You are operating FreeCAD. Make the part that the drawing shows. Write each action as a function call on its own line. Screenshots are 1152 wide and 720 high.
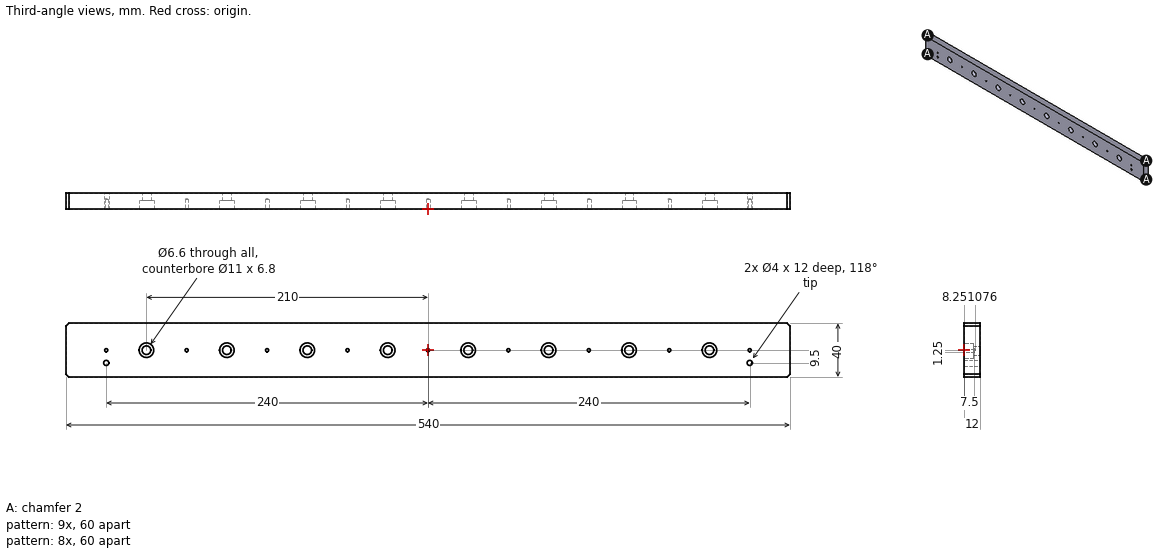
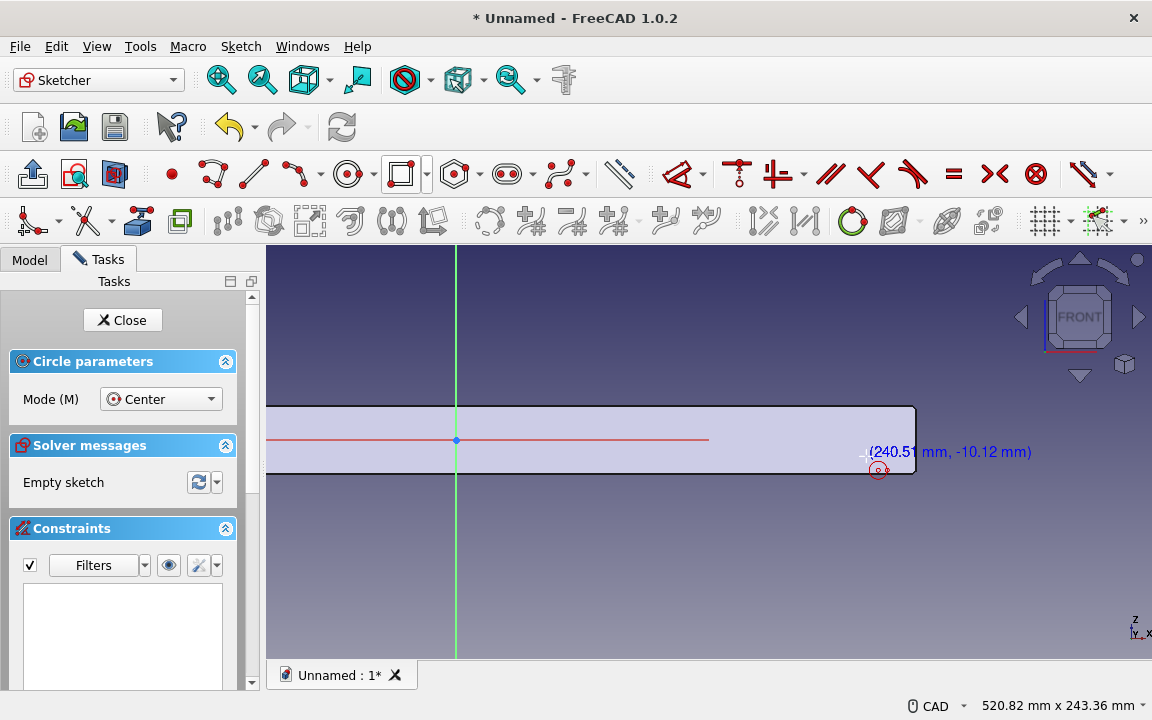
click(865, 456)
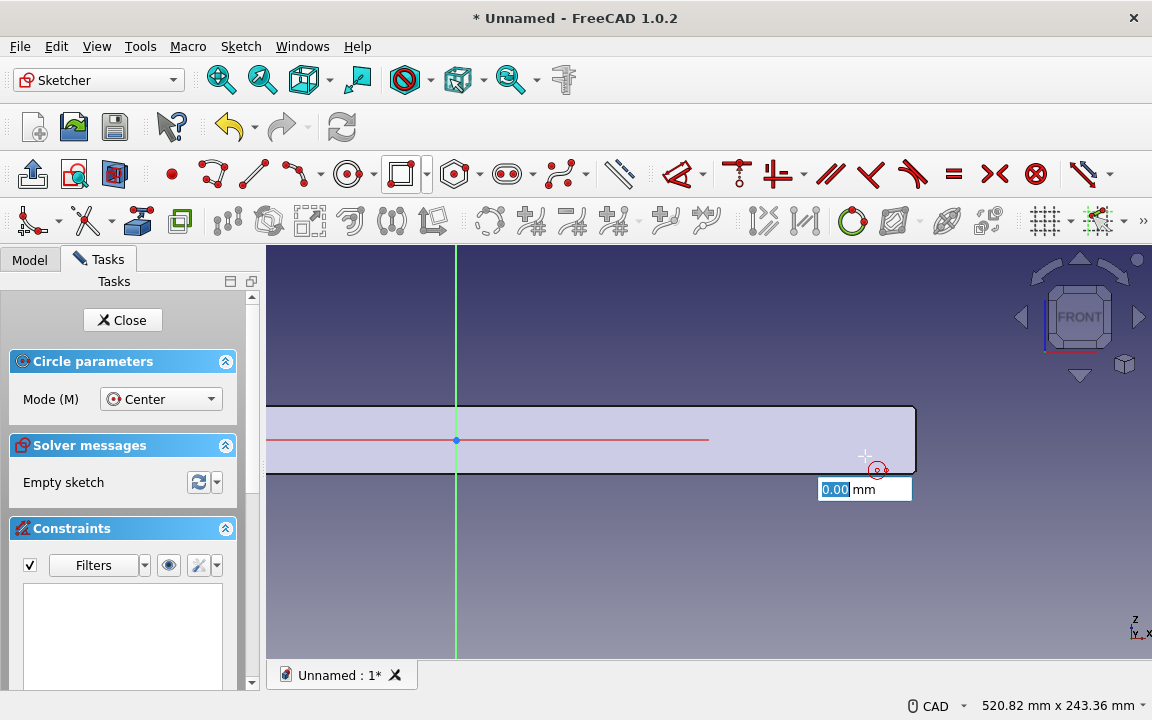
scroll(867, 459, up, 8)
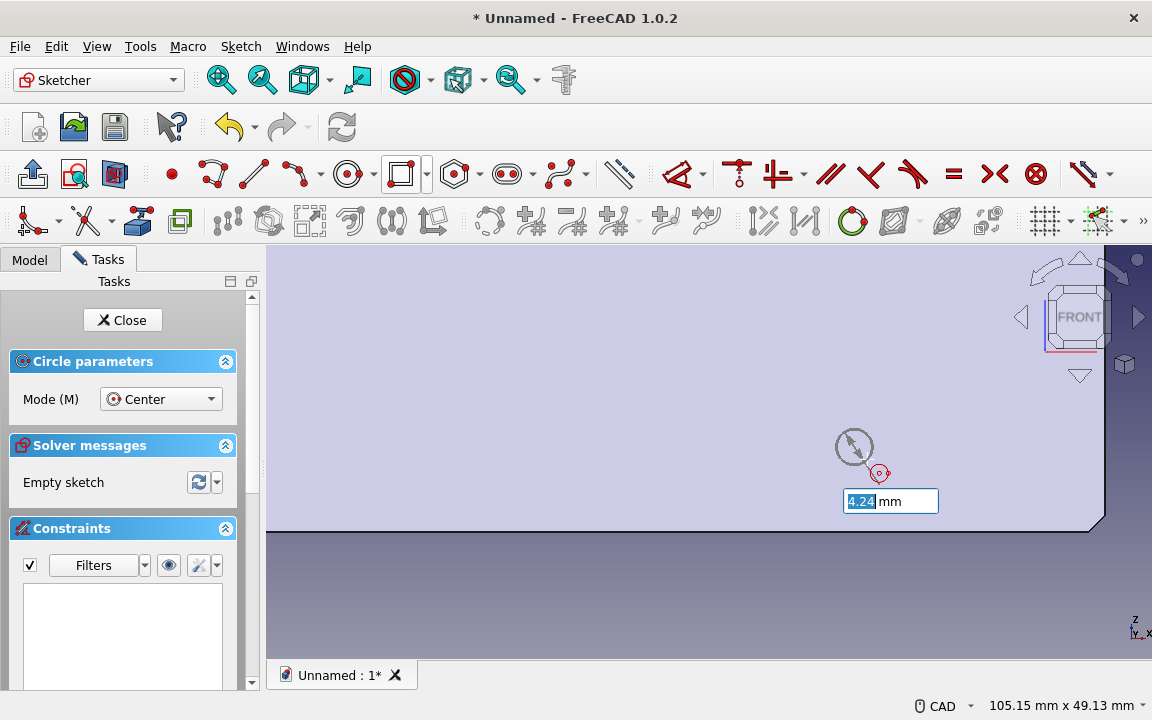
click(864, 456)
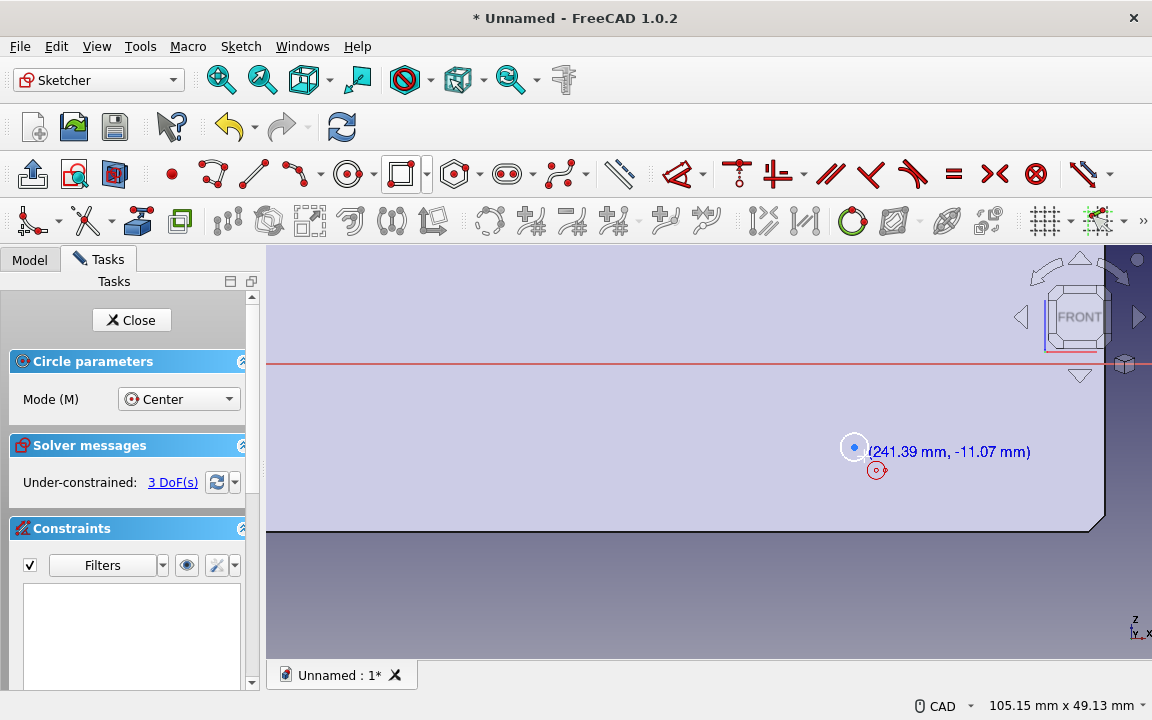
scroll(866, 457, down, 11)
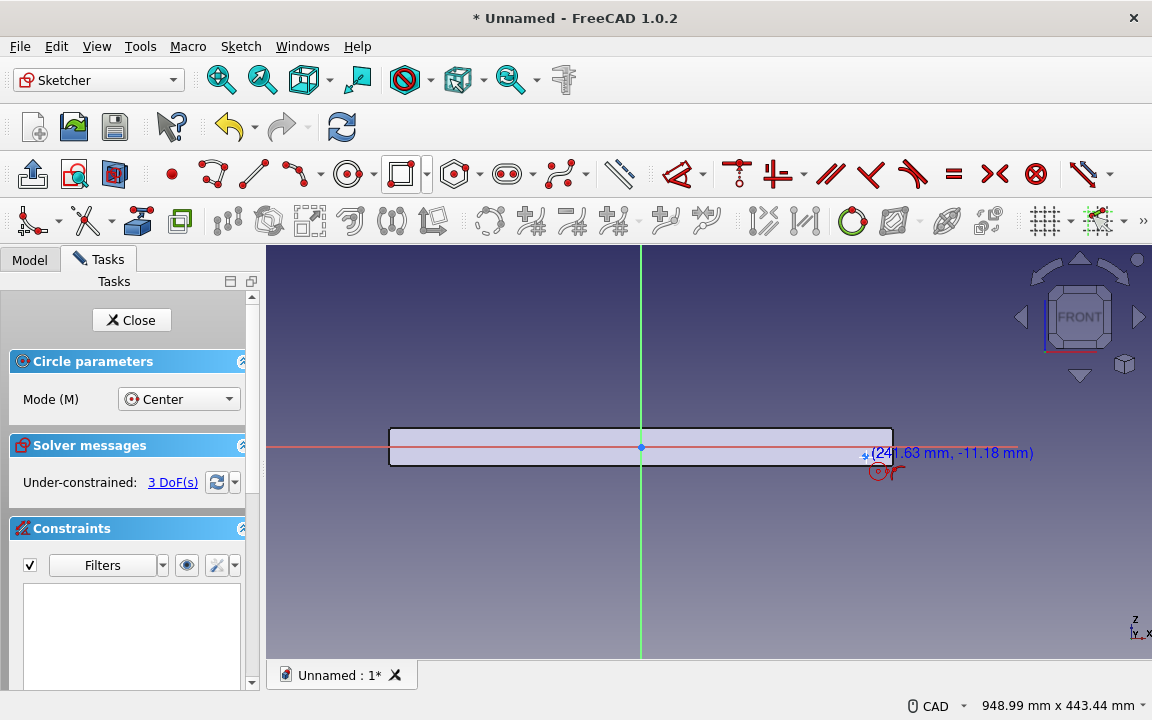
scroll(417, 456, up, 13)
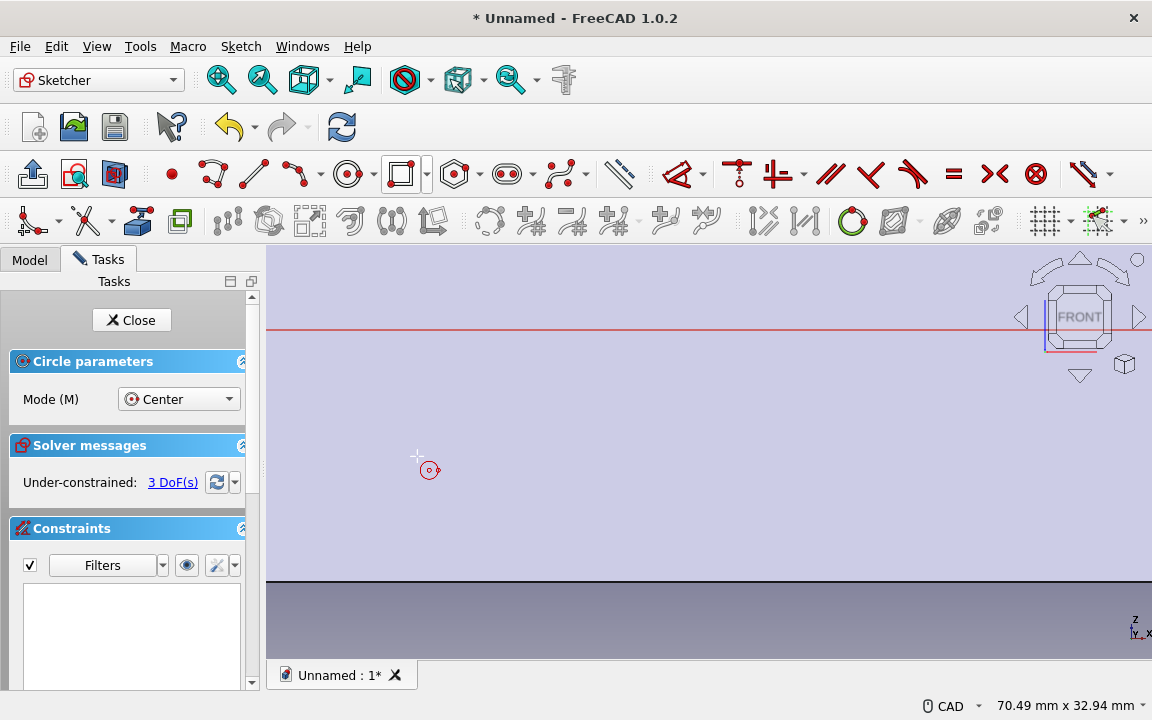
scroll(417, 456, down, 13)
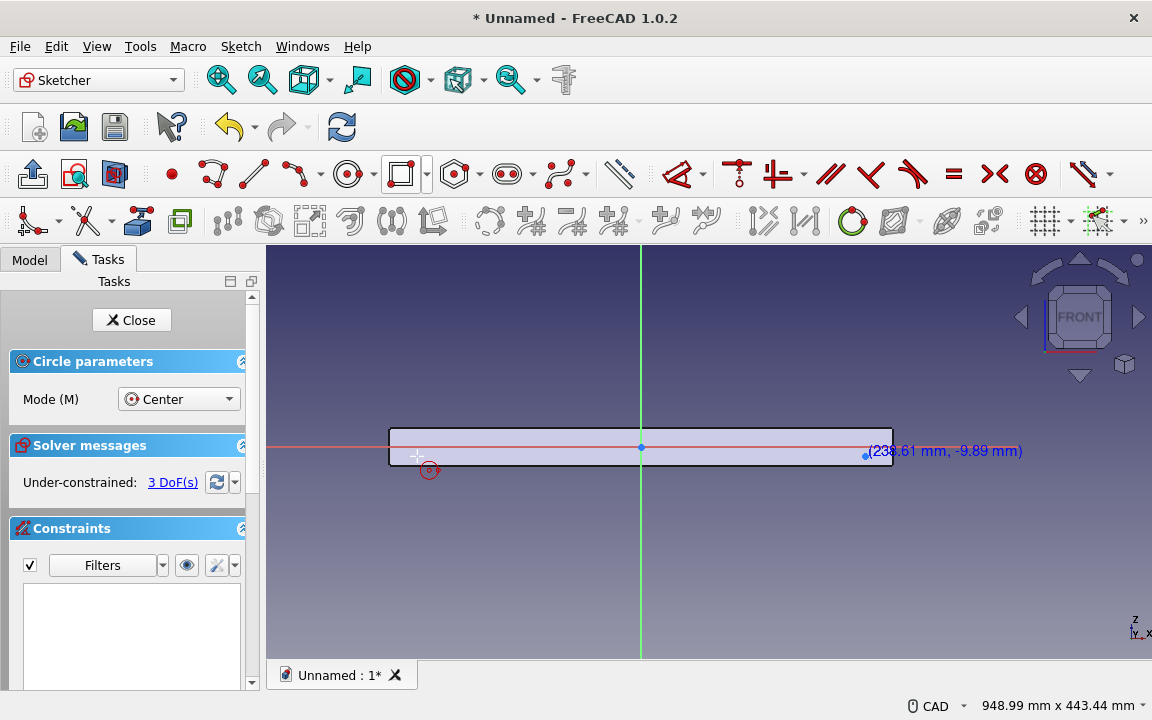
scroll(417, 456, up, 3)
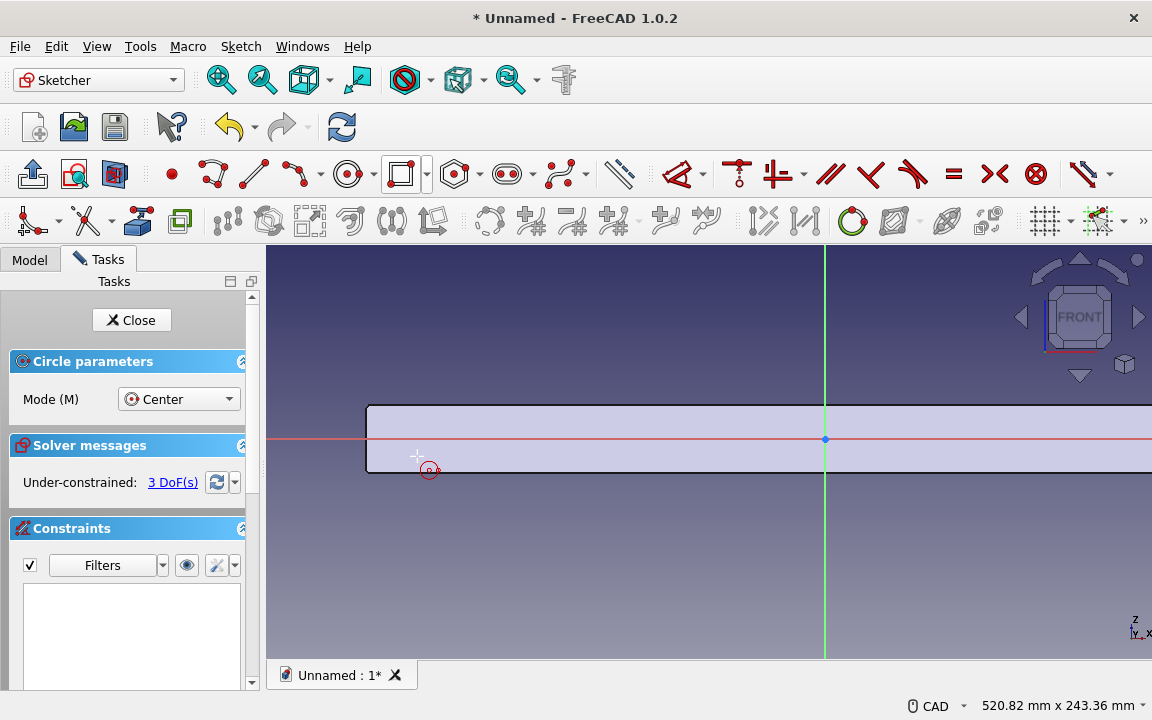
click(417, 456)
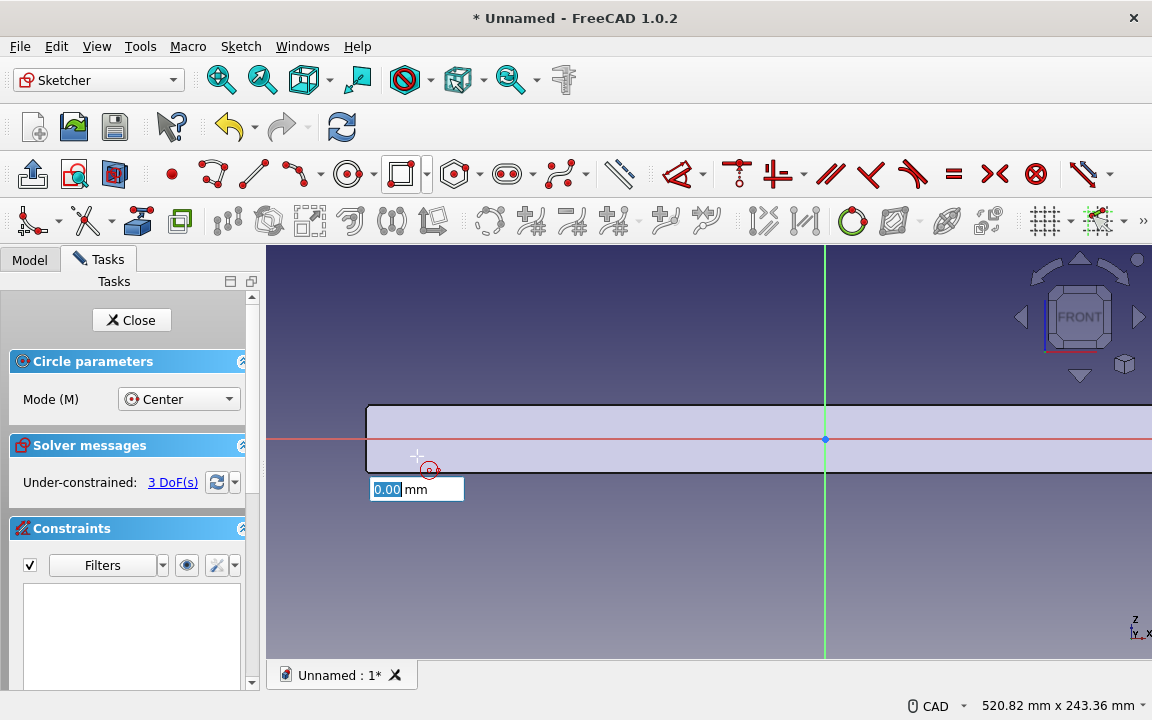
scroll(419, 458, up, 8)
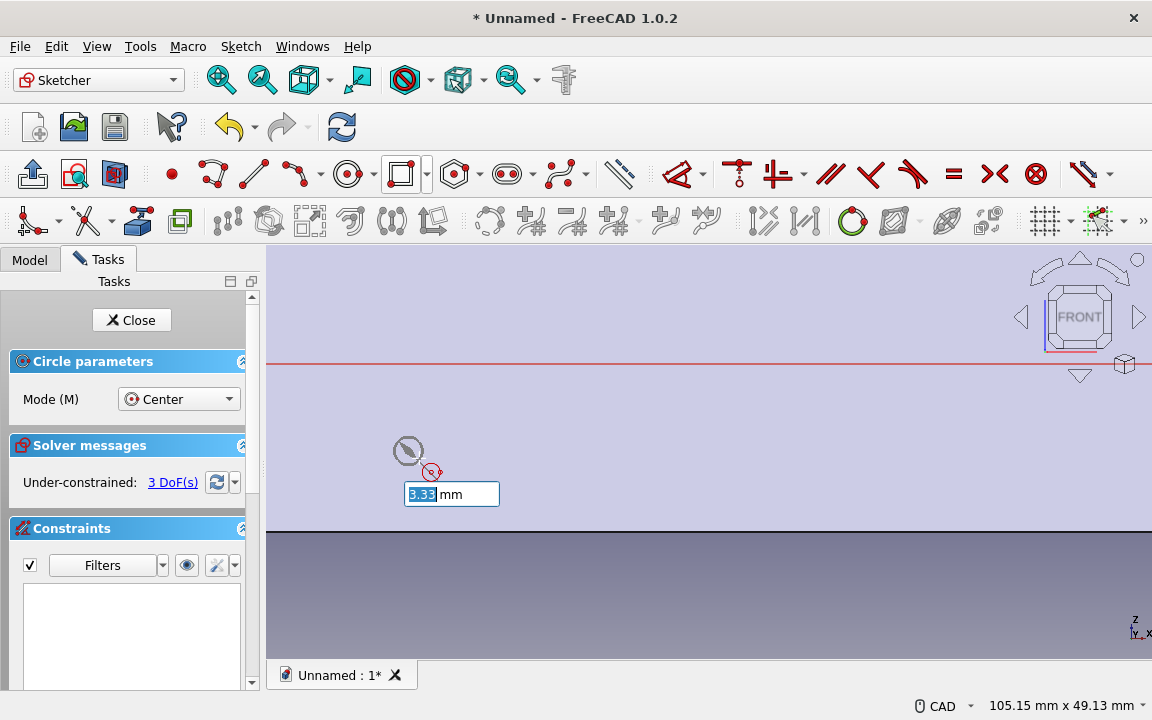
click(419, 456)
key(Escape)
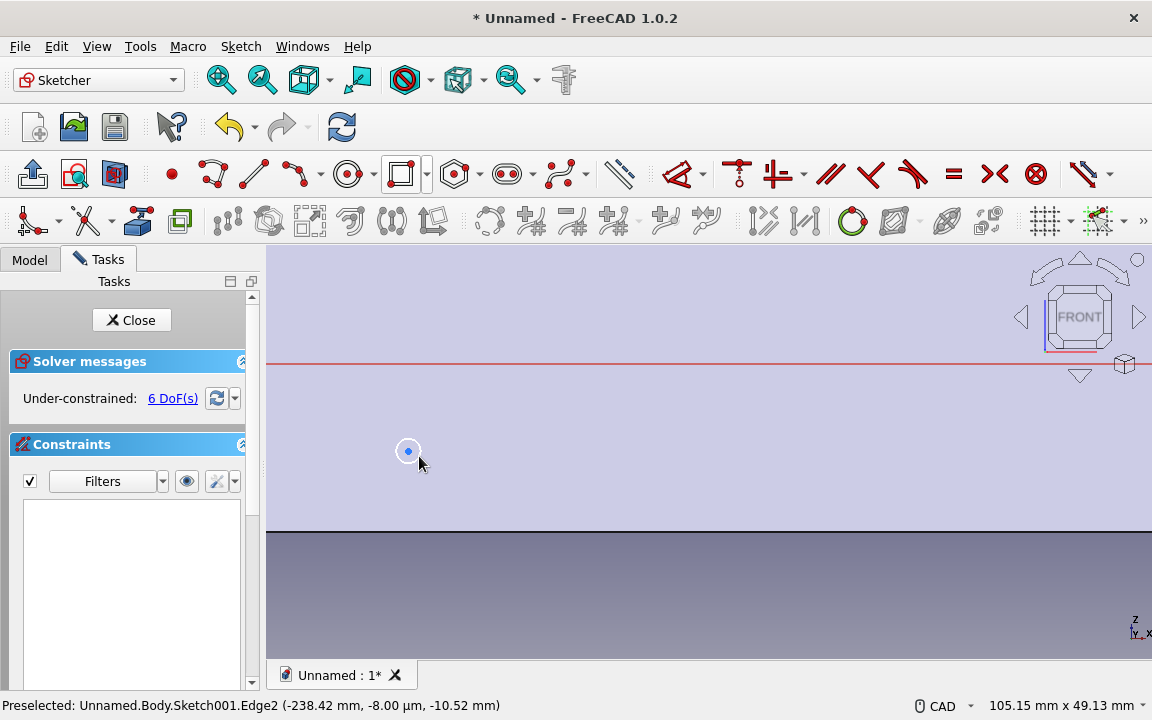
scroll(418, 457, down, 11)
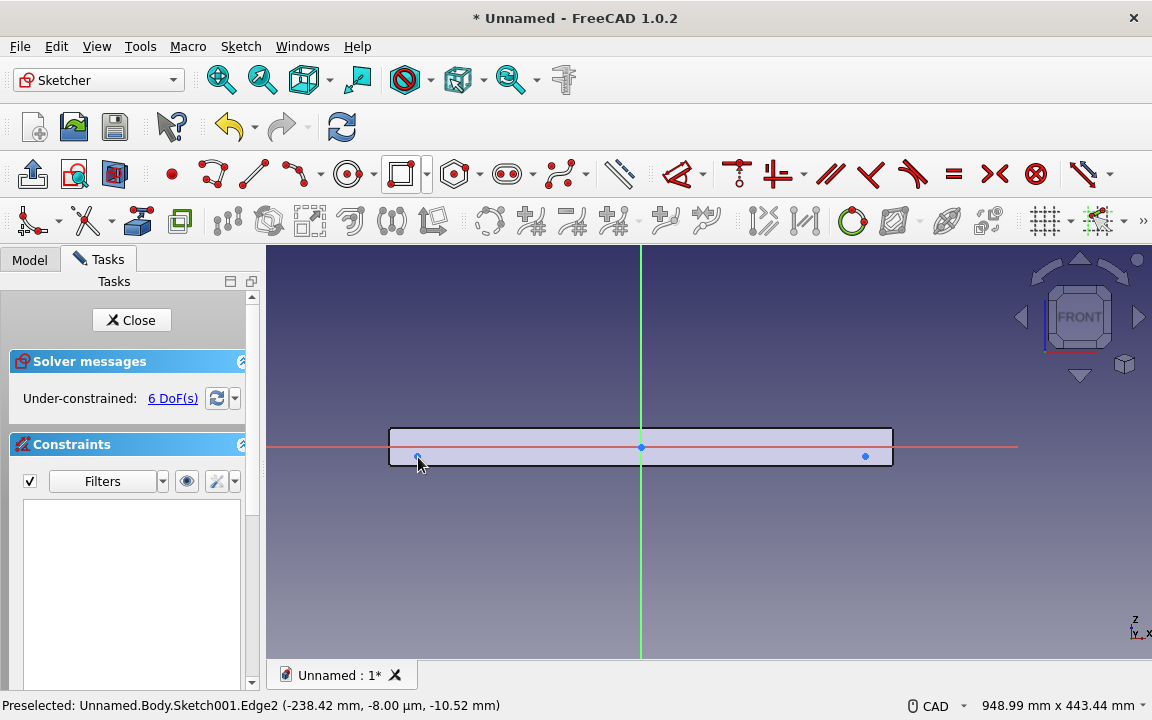
scroll(866, 455, up, 11)